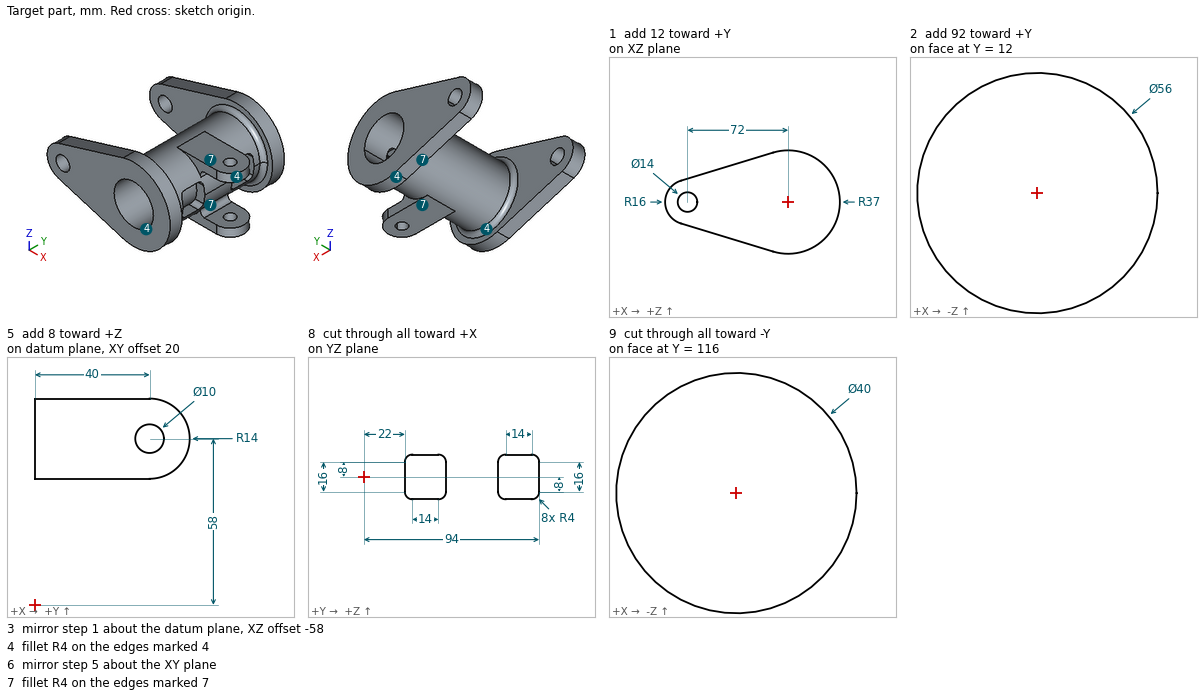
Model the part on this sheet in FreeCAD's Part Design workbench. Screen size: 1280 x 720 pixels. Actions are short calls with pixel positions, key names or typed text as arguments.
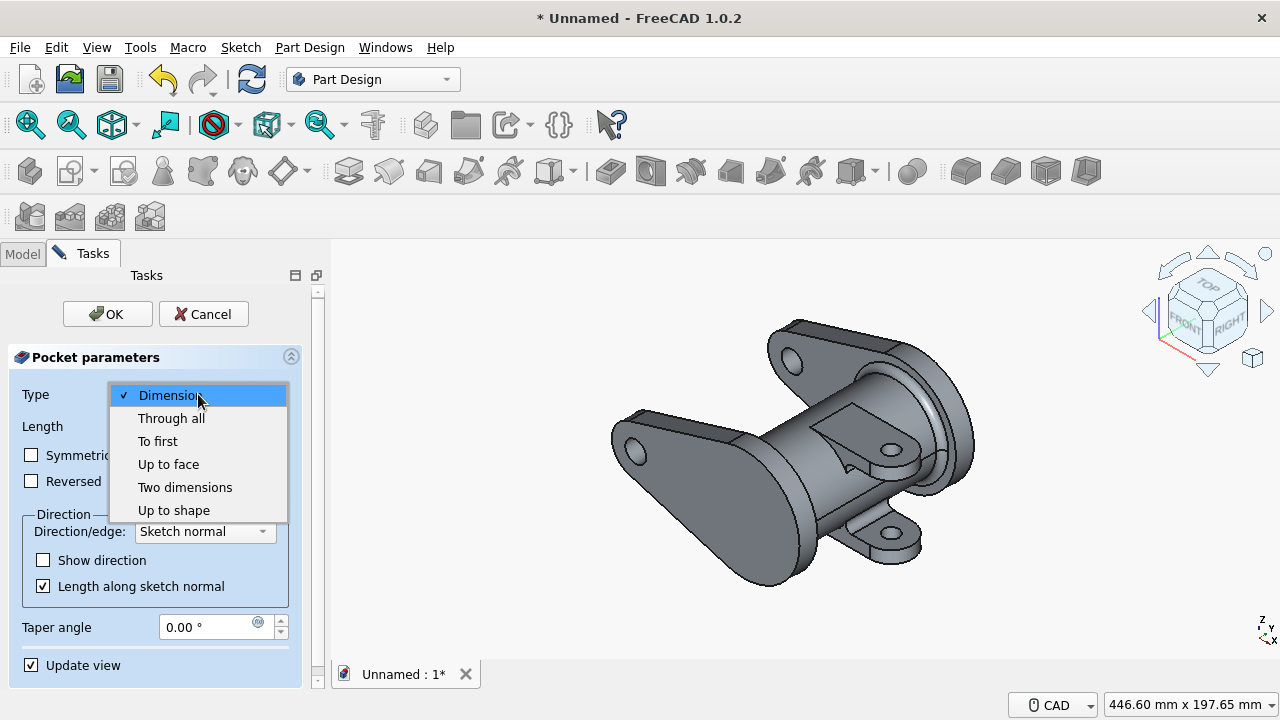
click(198, 418)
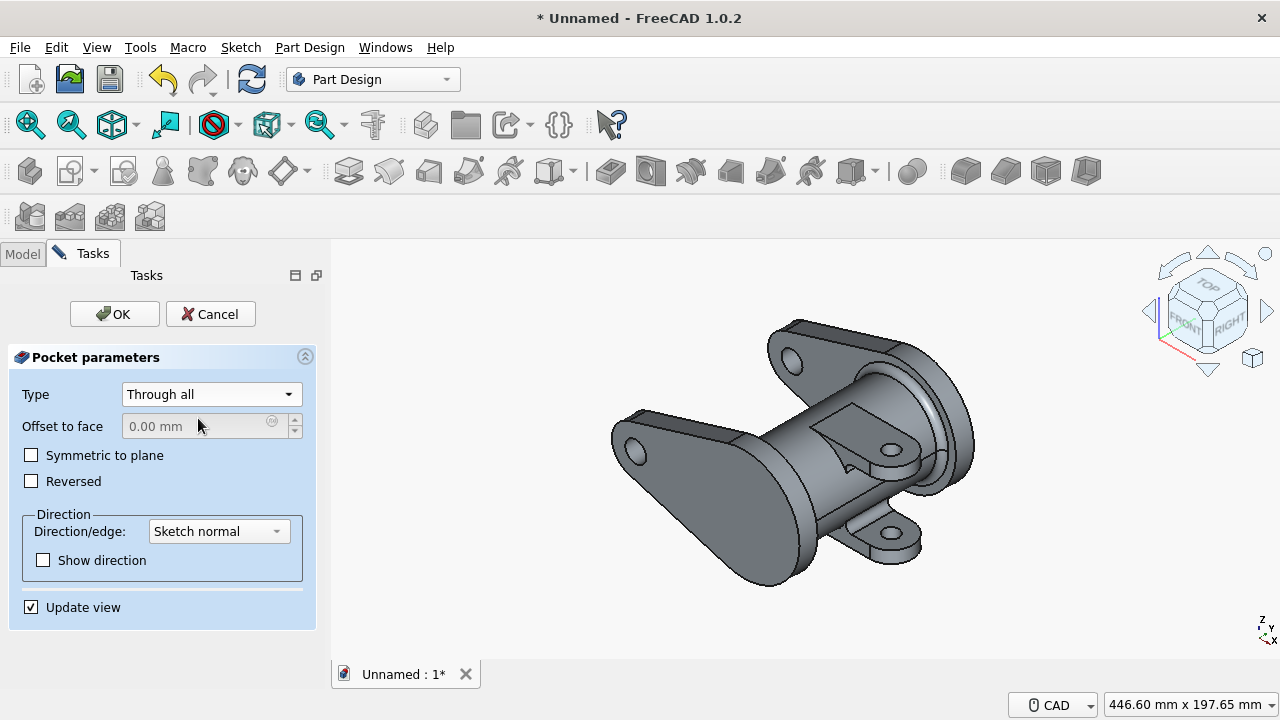
click(30, 481)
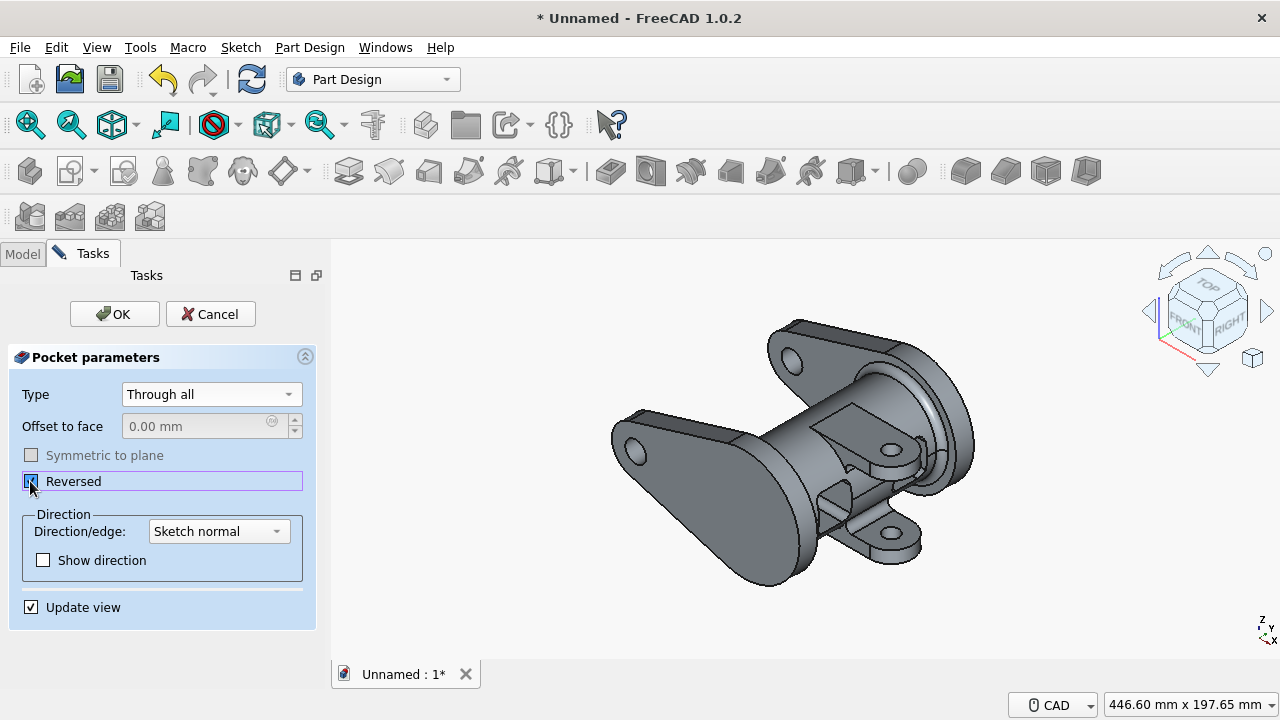
click(115, 314)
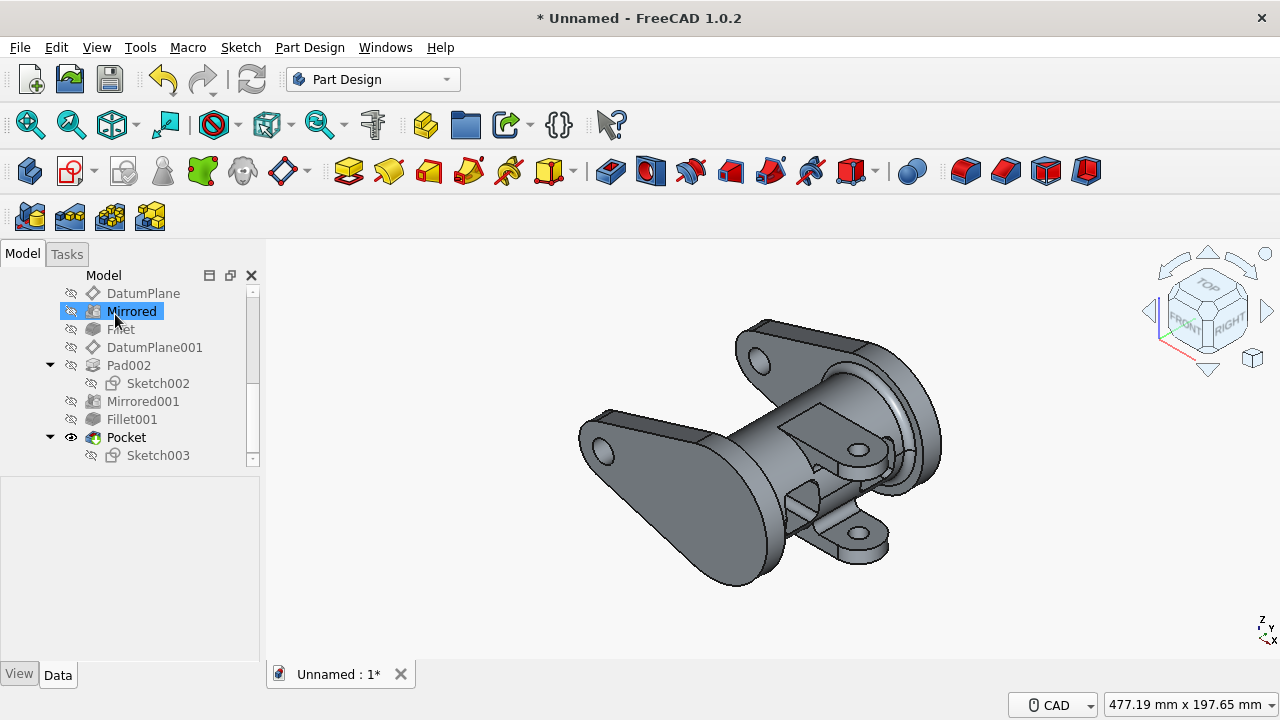
key(4)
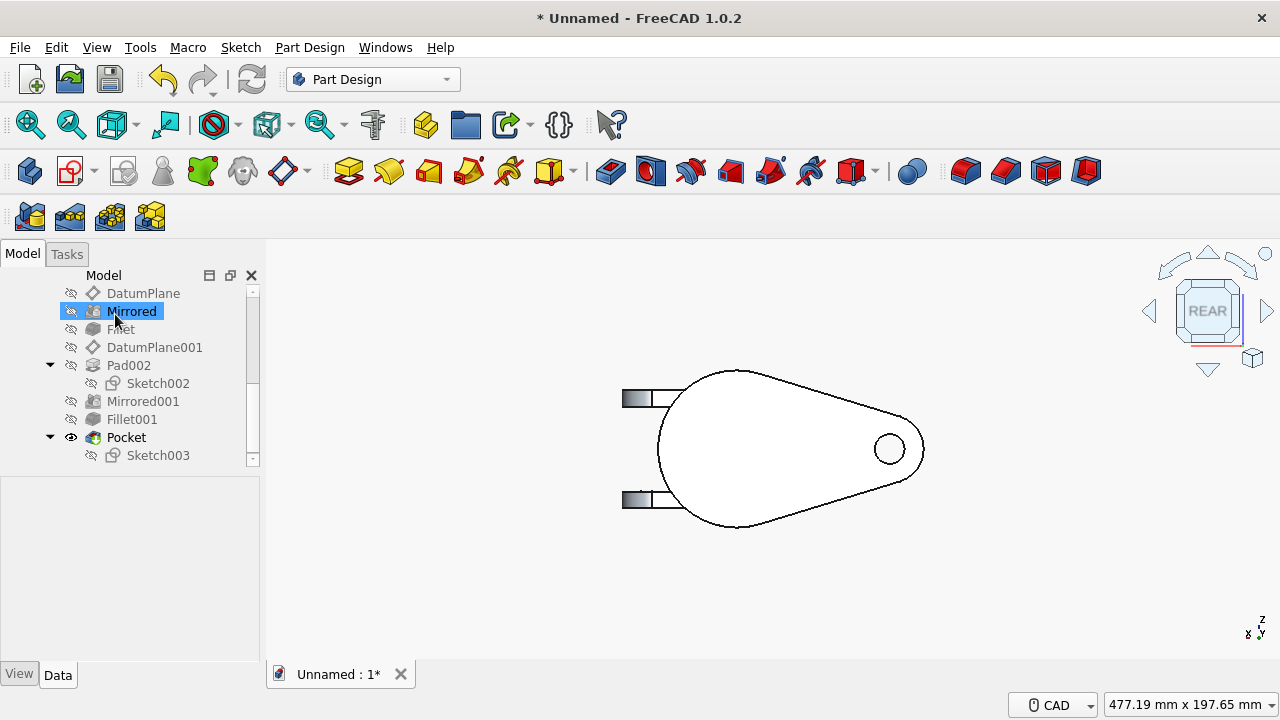
click(32, 126)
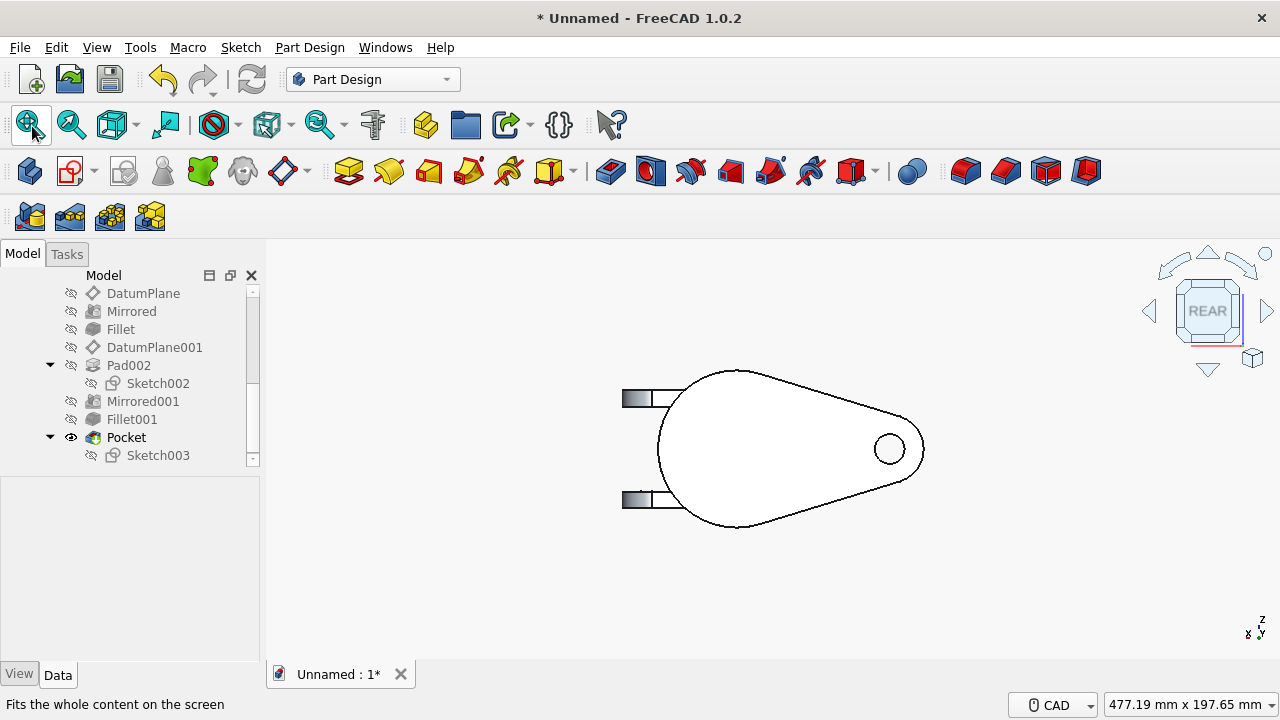
click(753, 448)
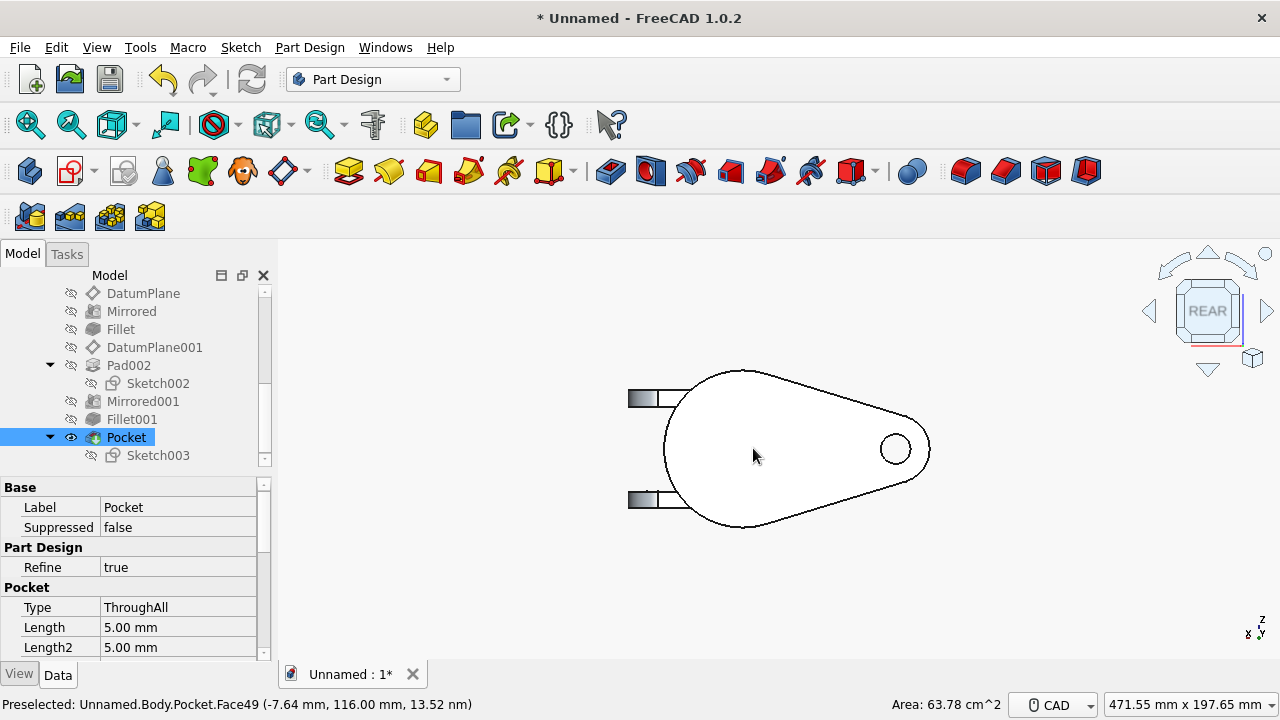
click(70, 172)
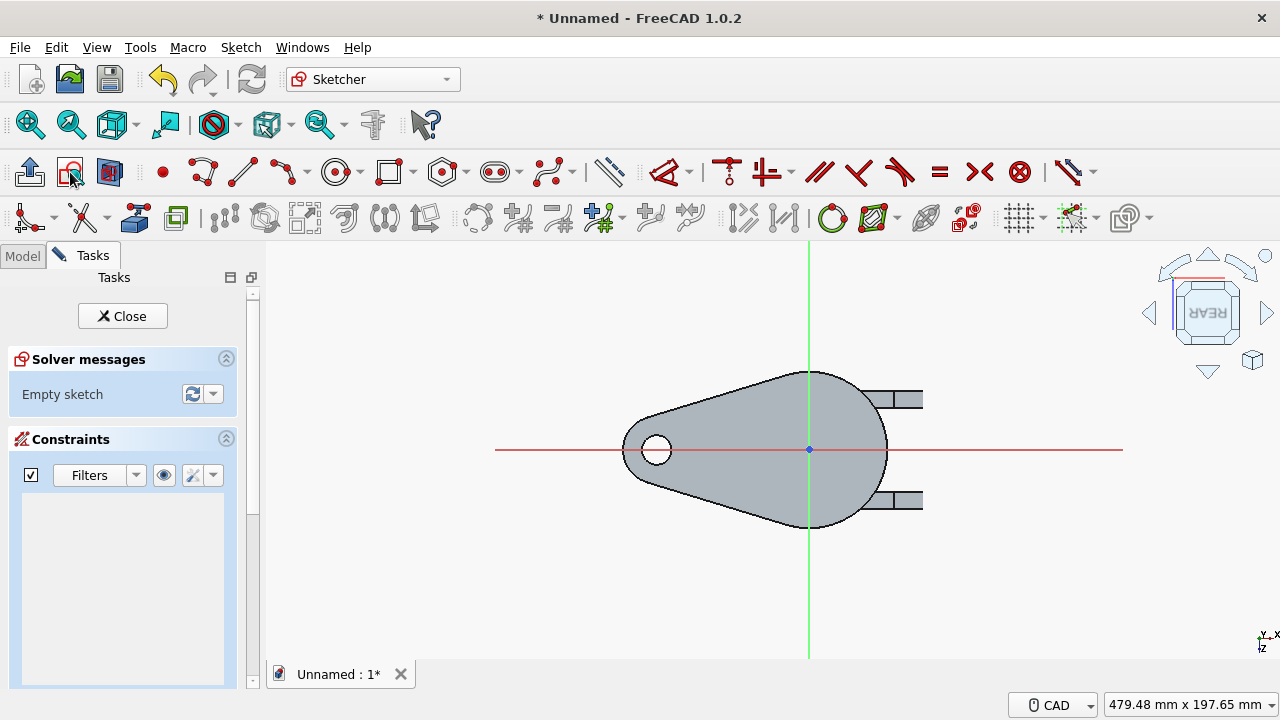
scroll(854, 450, up, 6)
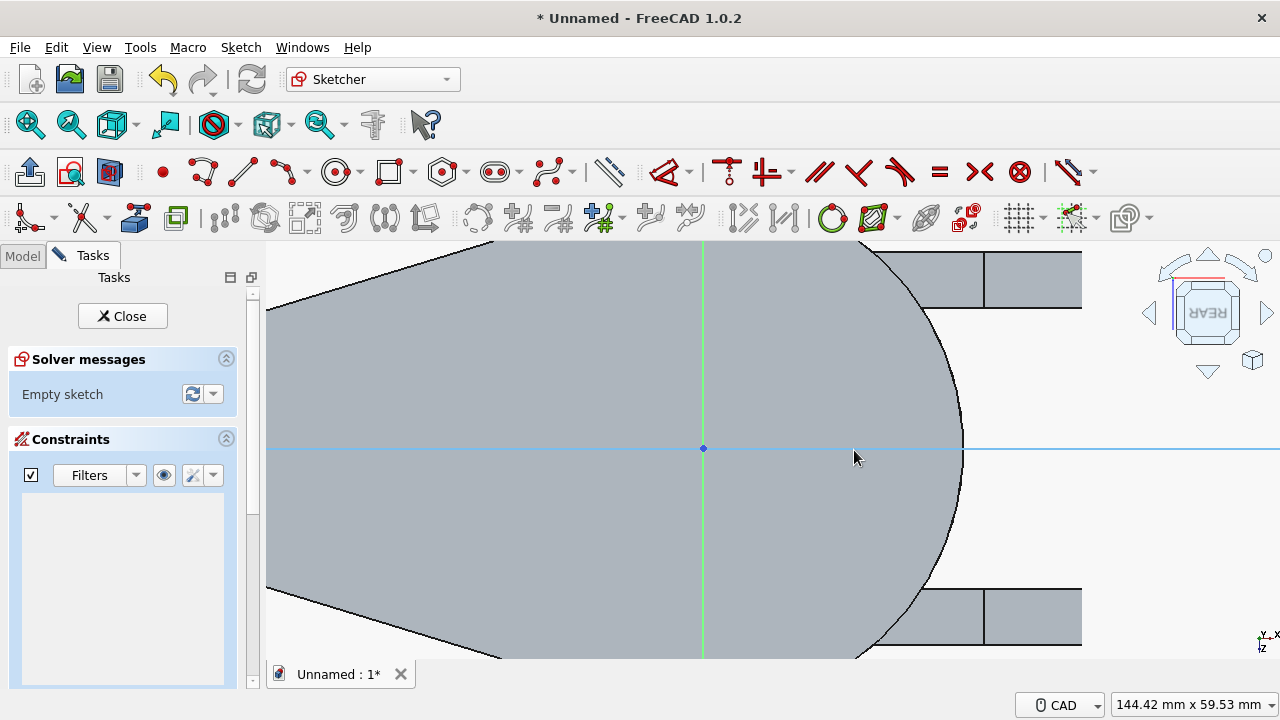
click(336, 172)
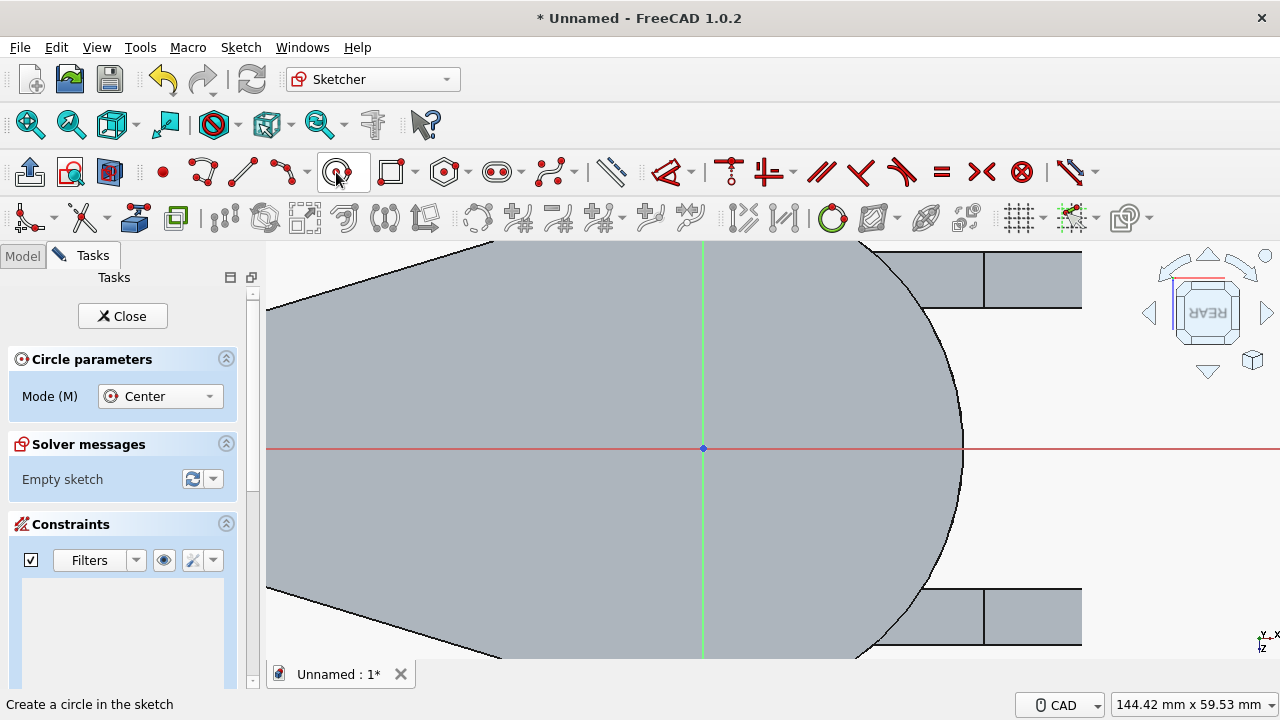
click(703, 449)
move(803, 350)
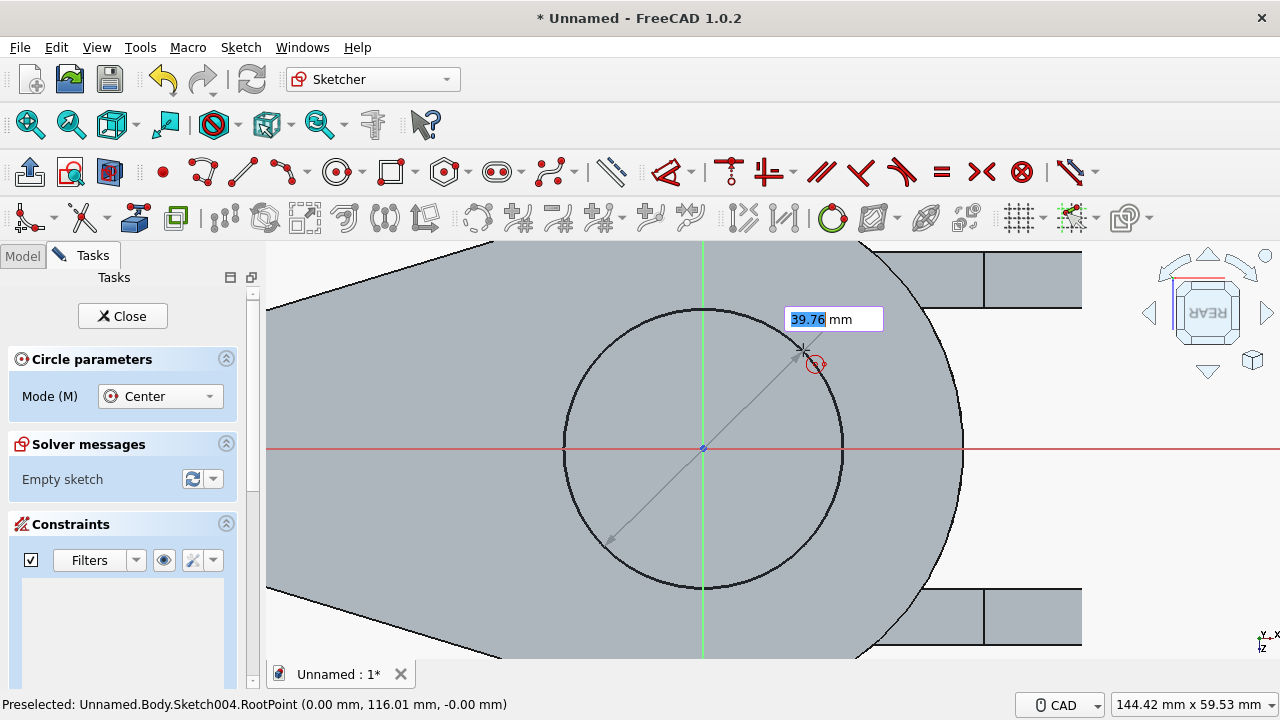
text(40)
key(Return)
key(Escape)